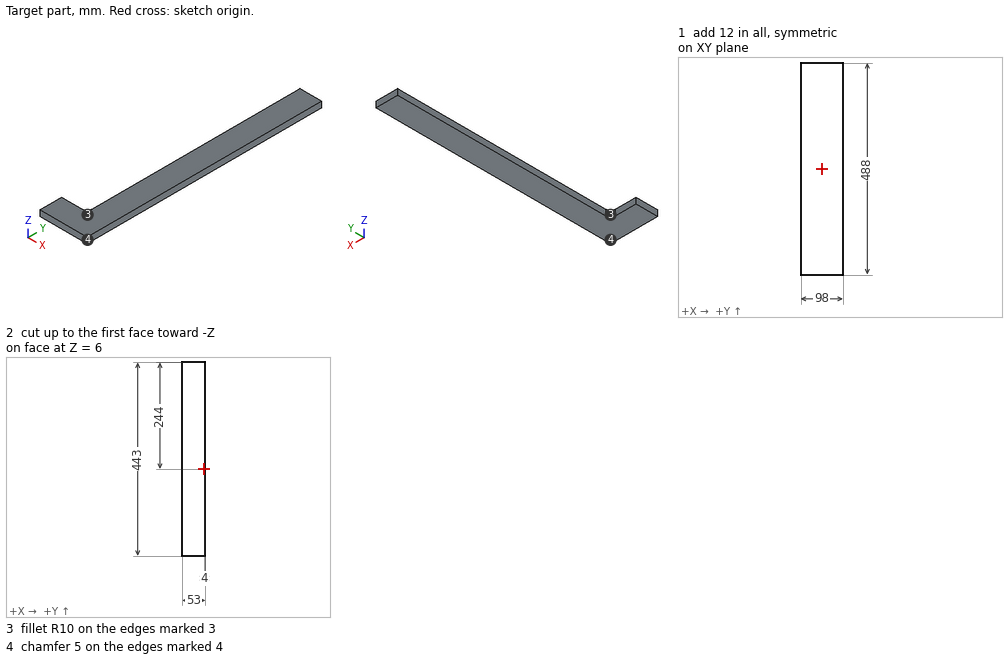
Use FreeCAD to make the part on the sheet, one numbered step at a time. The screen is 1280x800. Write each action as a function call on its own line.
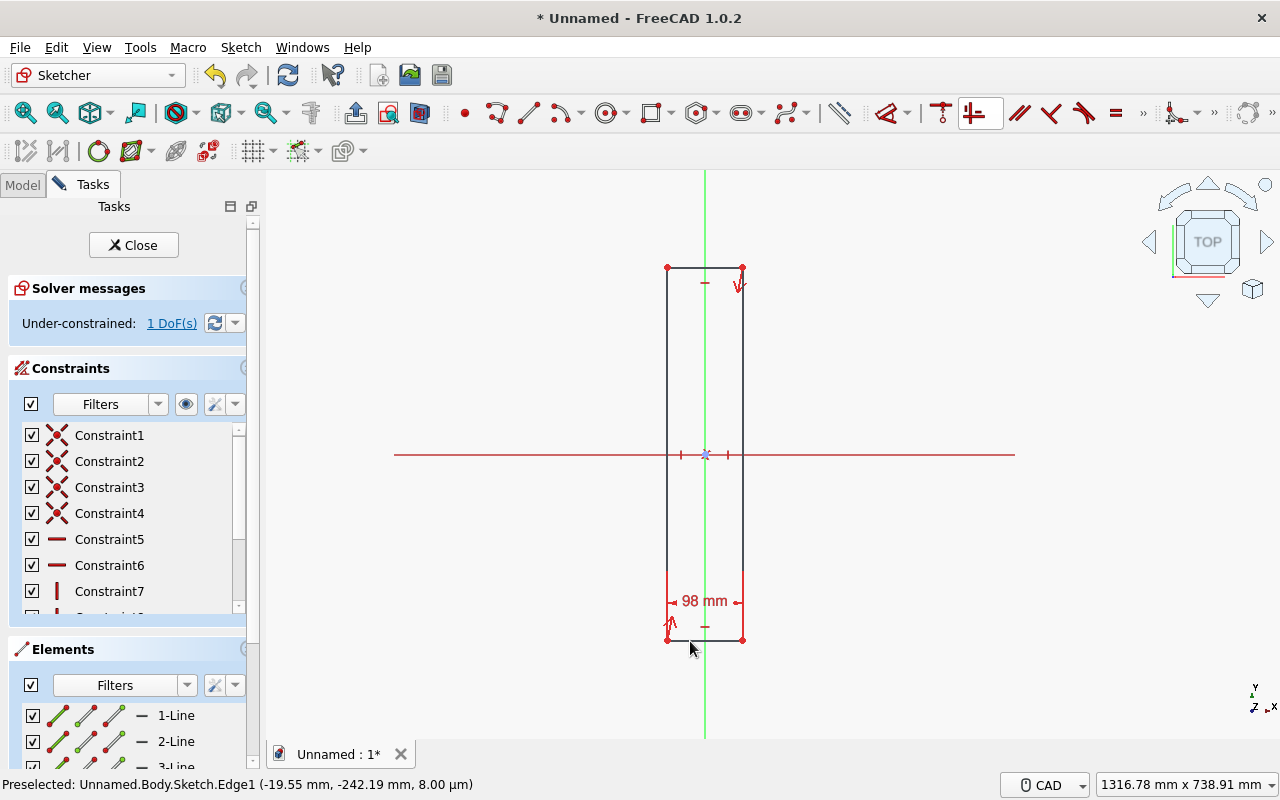
click(743, 529)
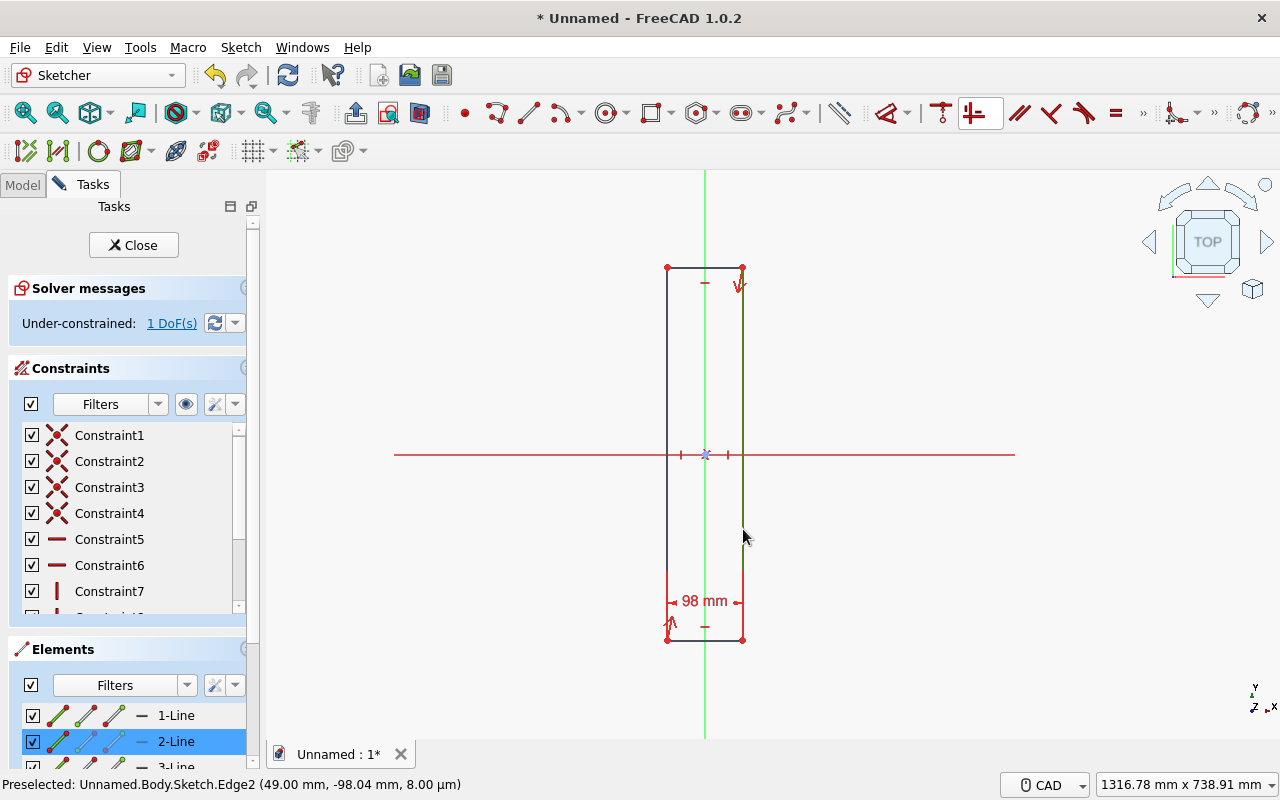
key(i)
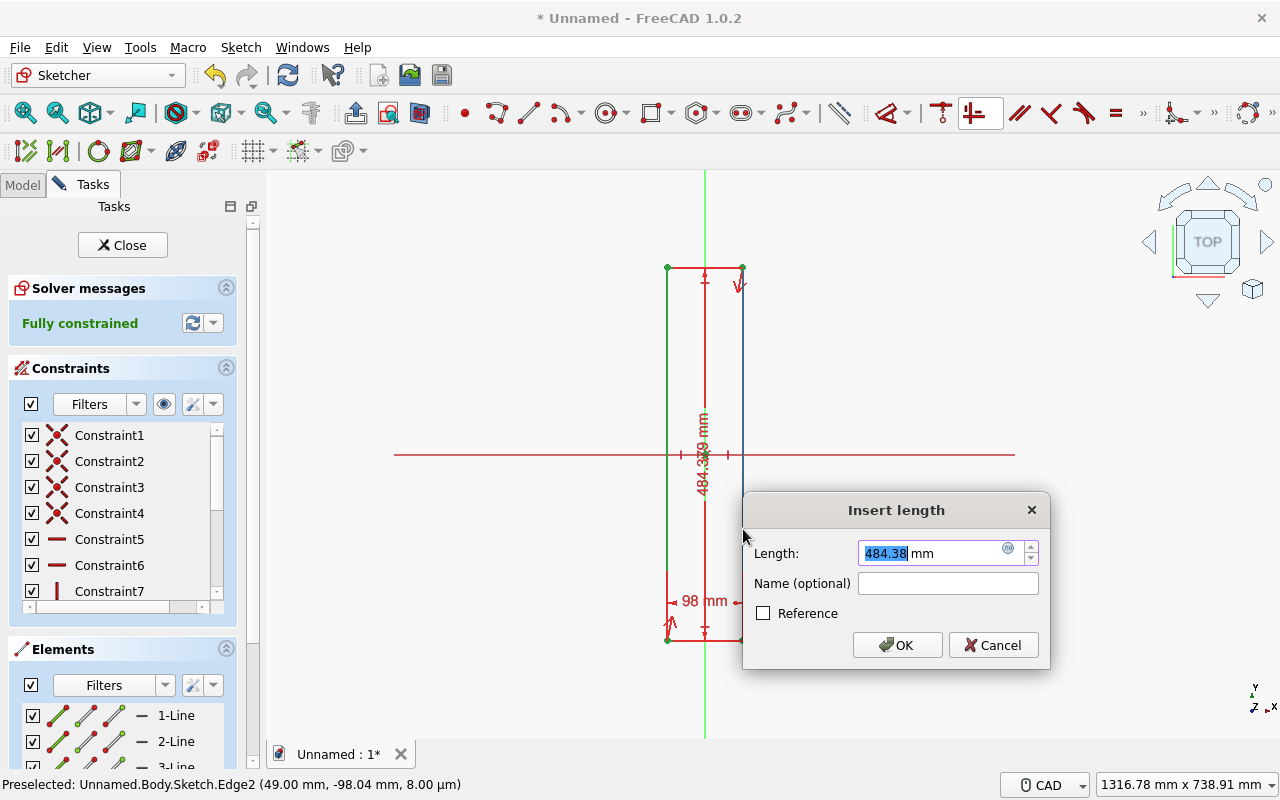
text(488)
key(Return)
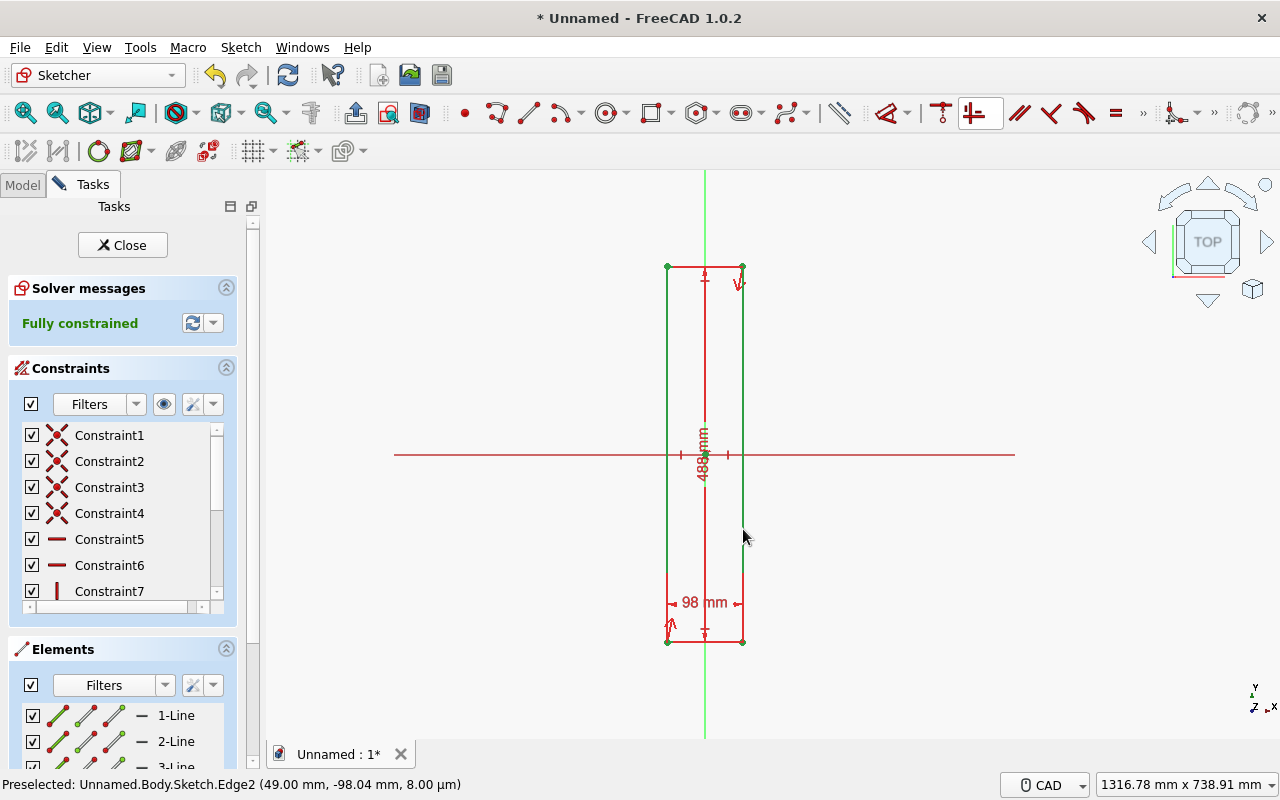
click(123, 245)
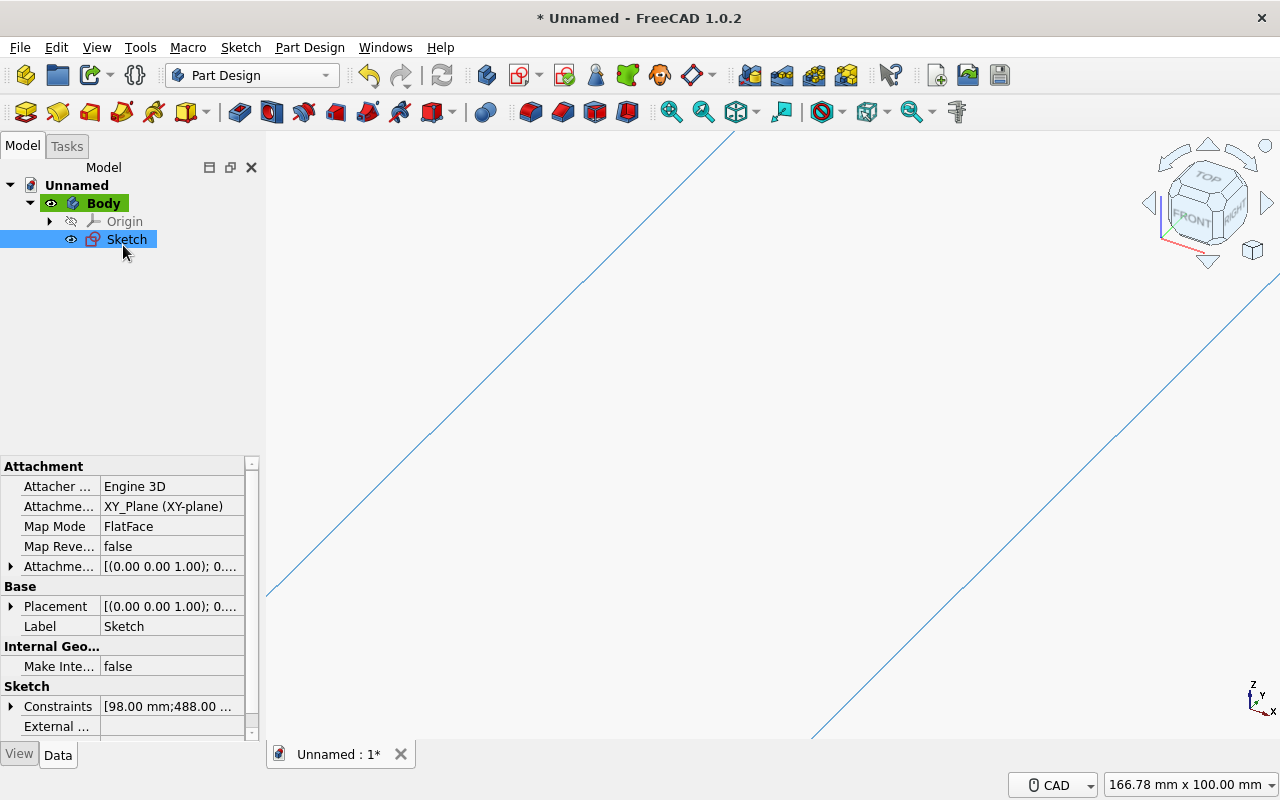
click(26, 112)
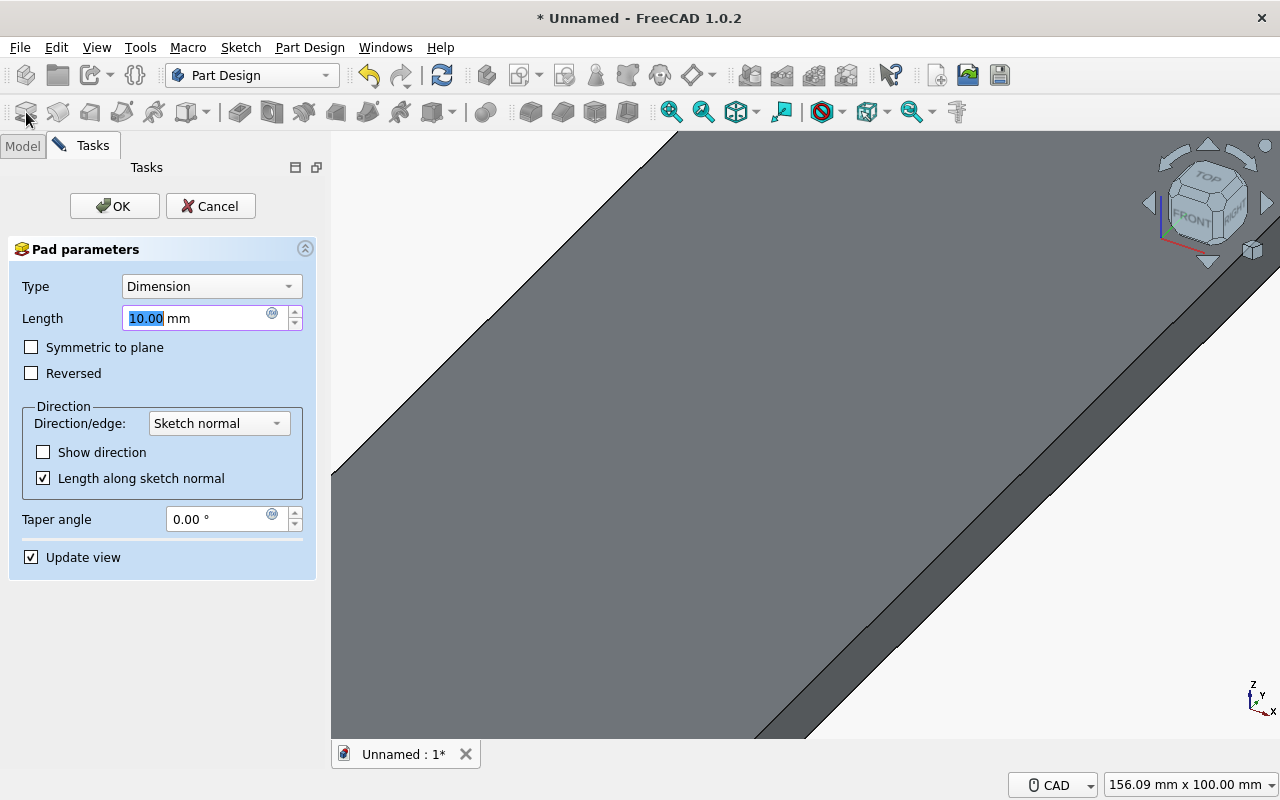
text(12)
key(Tab)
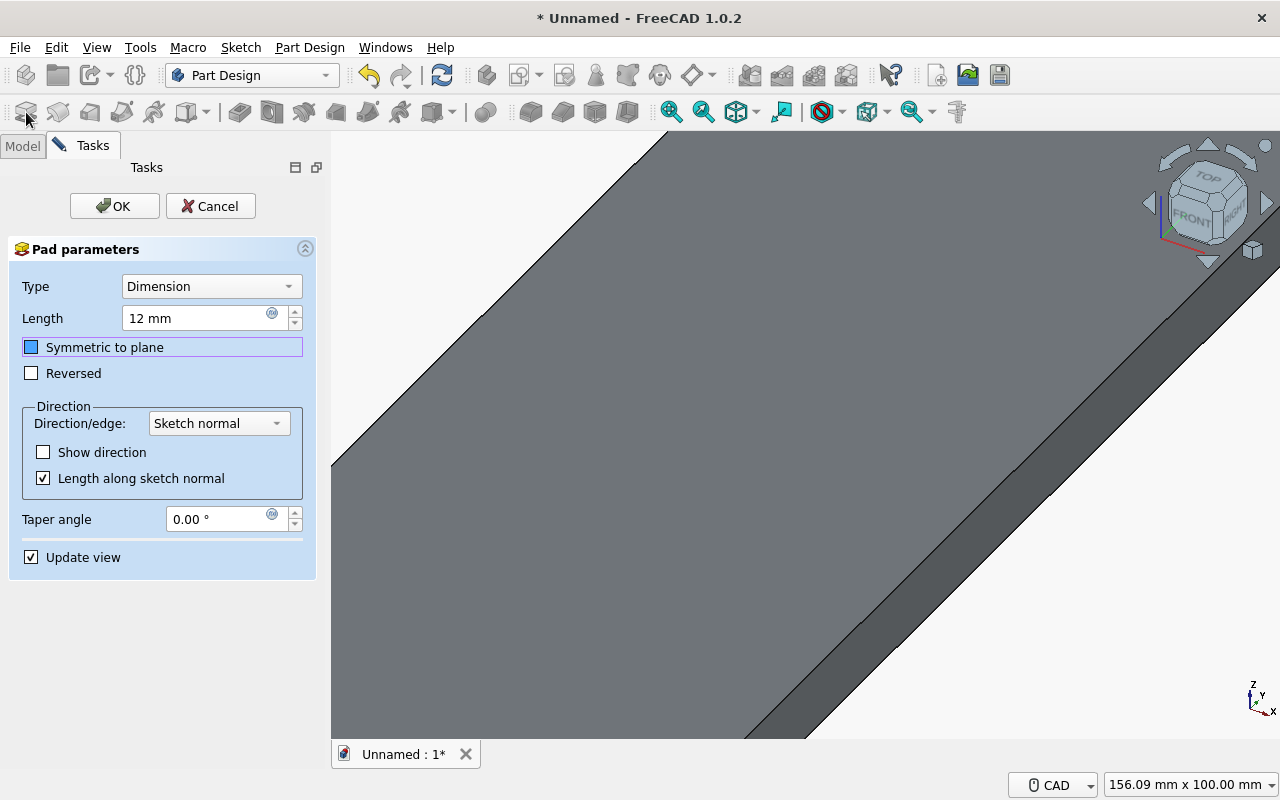
click(30, 347)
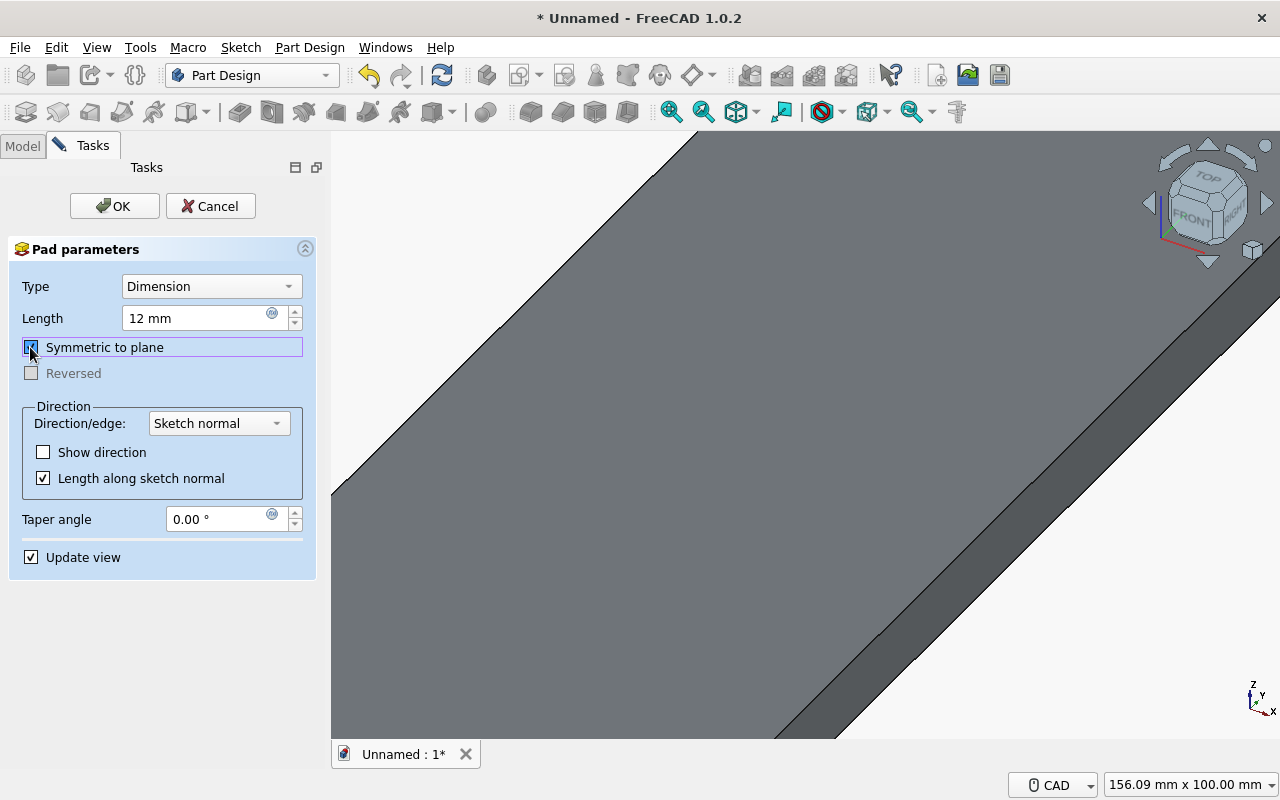
click(115, 206)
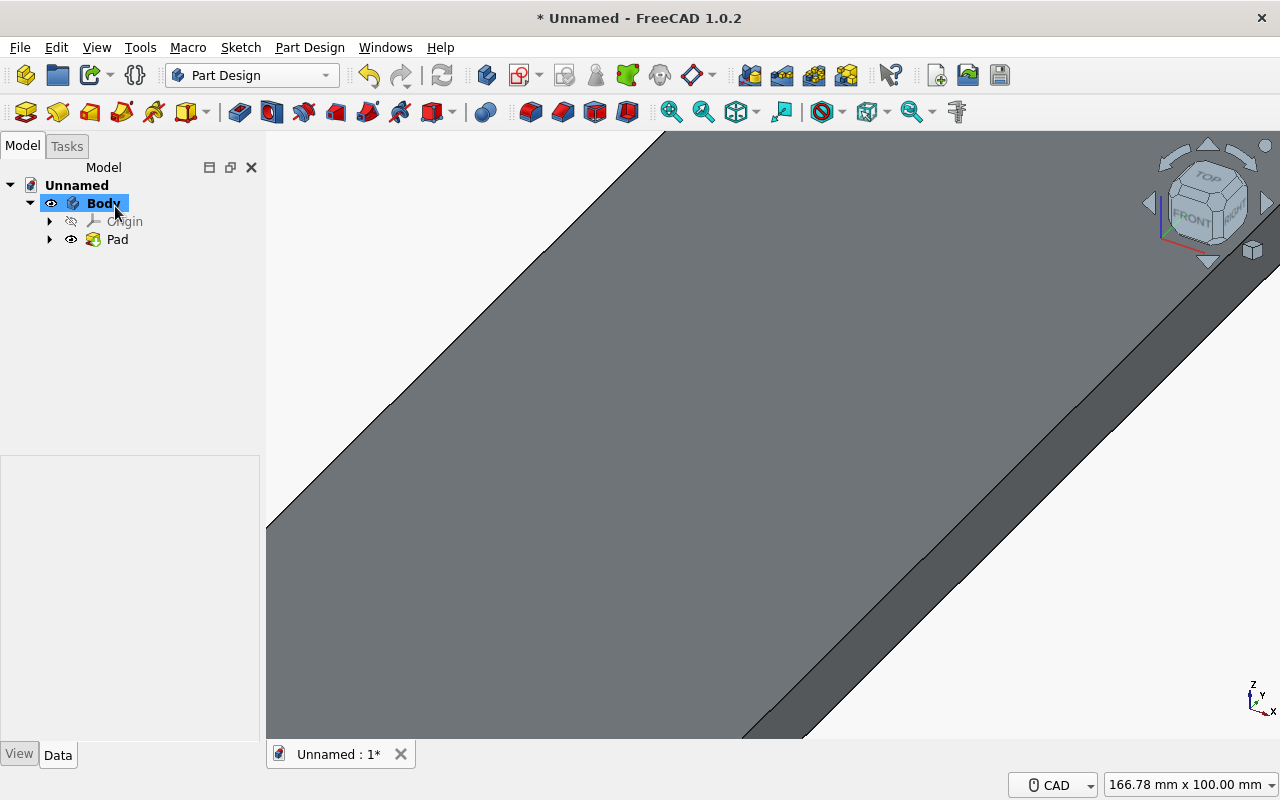
key(v)
key(f)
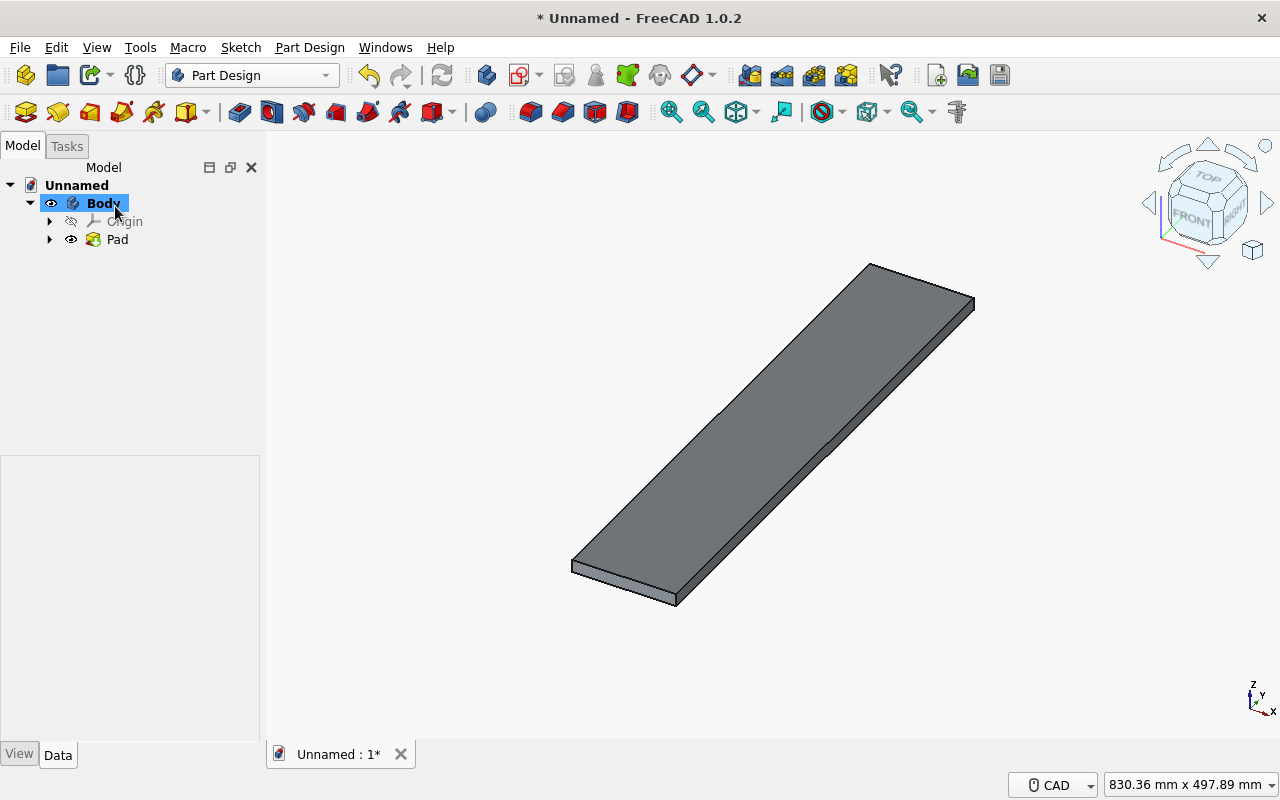
click(858, 343)